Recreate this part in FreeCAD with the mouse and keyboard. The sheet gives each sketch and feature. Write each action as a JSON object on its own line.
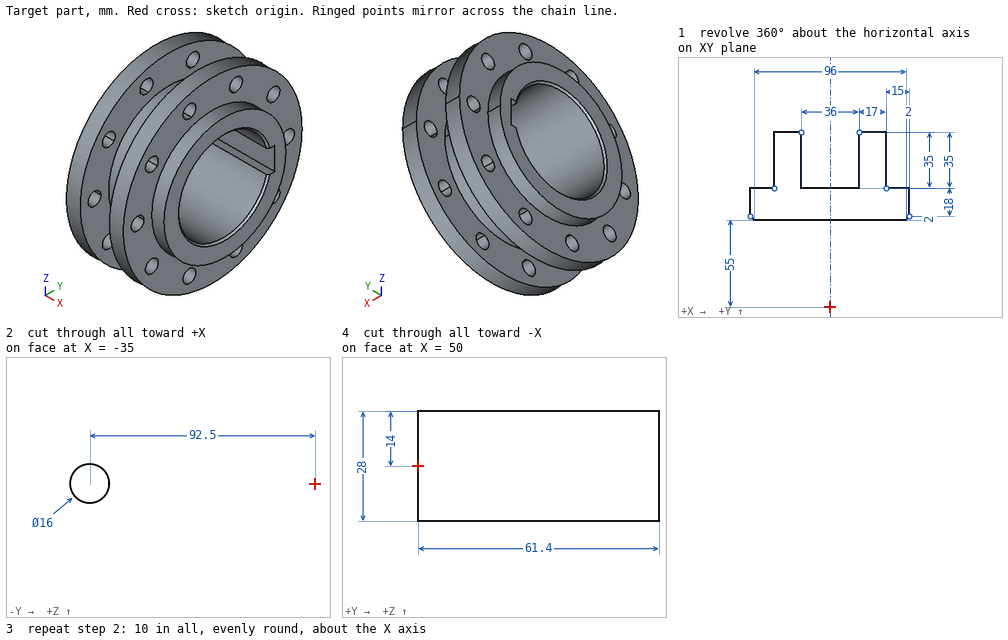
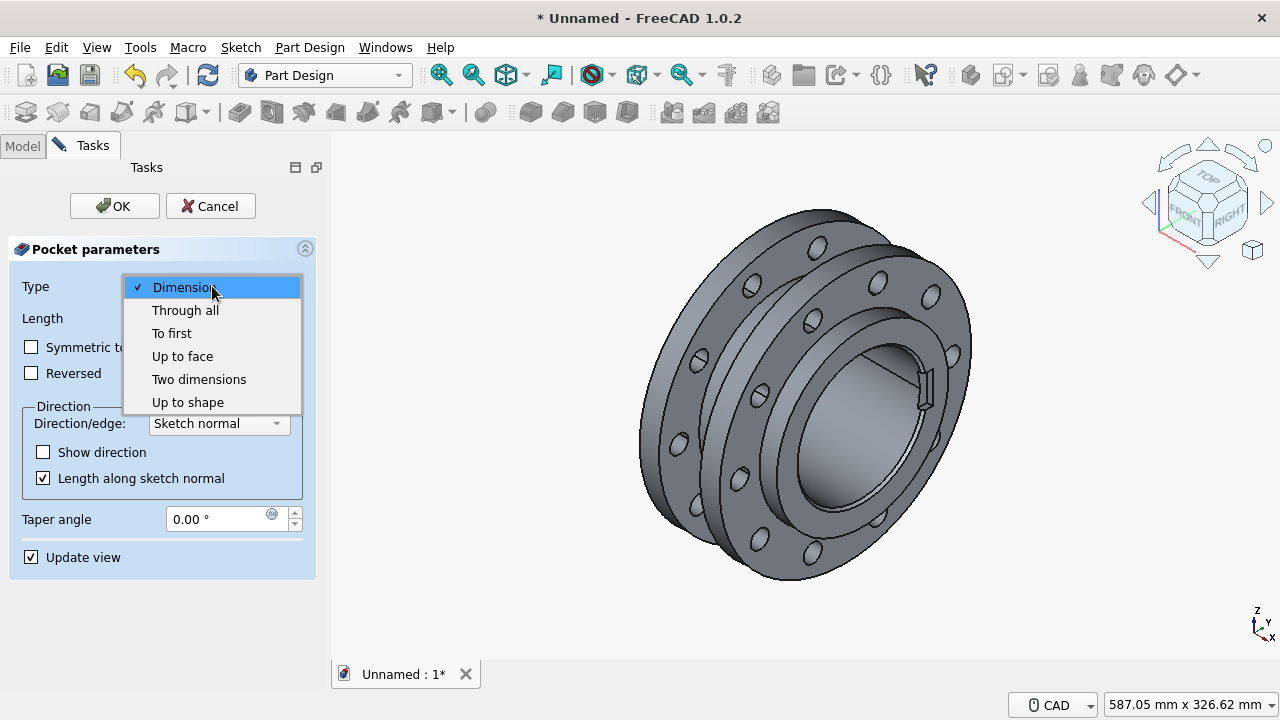
{"action": "left_click", "coordinate": [212, 310]}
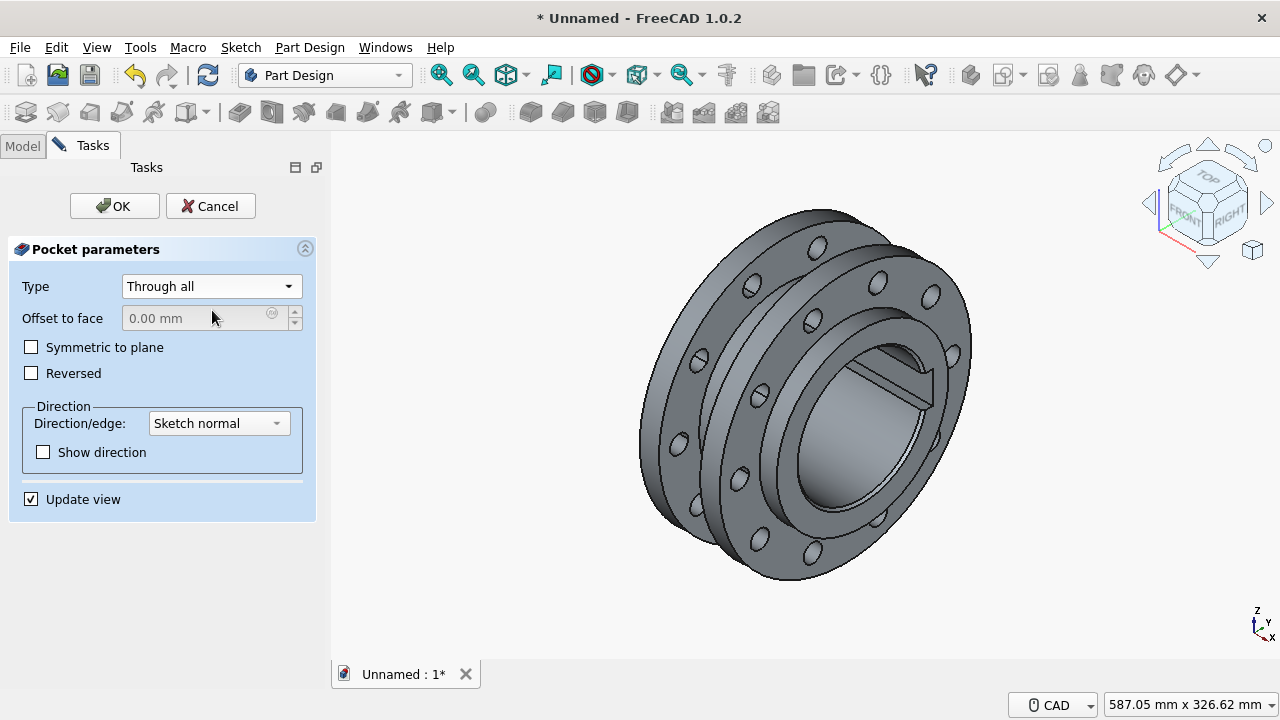
{"action": "left_click", "coordinate": [115, 206]}